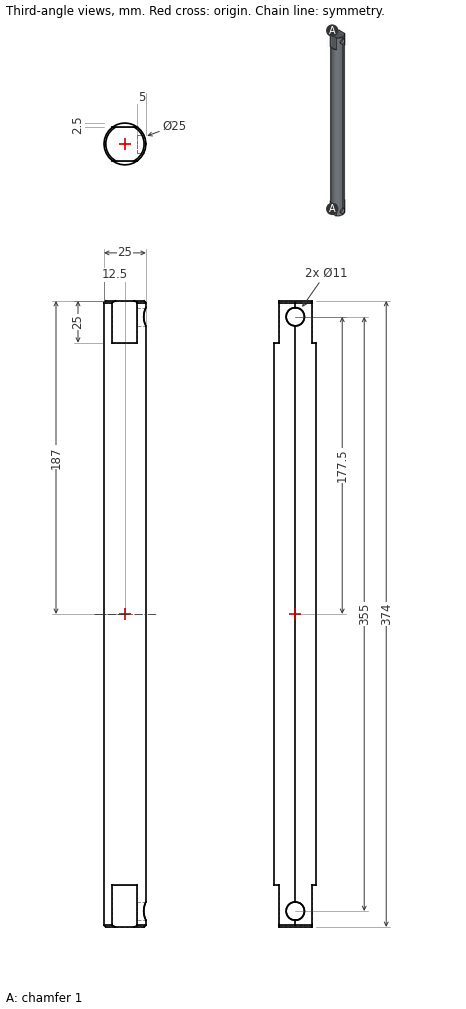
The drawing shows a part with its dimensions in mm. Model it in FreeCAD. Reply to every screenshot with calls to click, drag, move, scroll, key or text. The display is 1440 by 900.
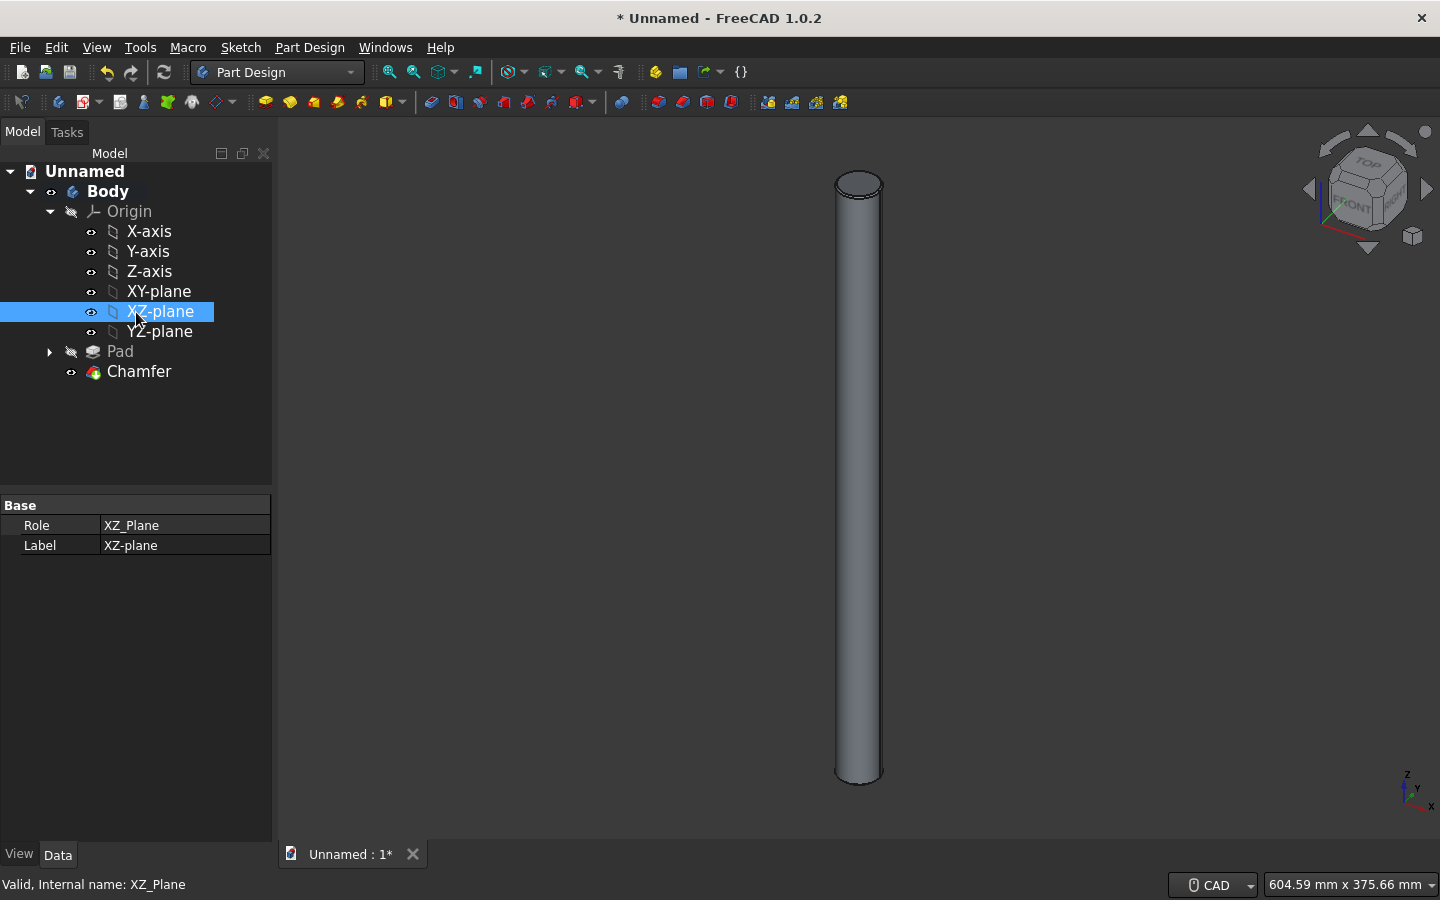
click(216, 102)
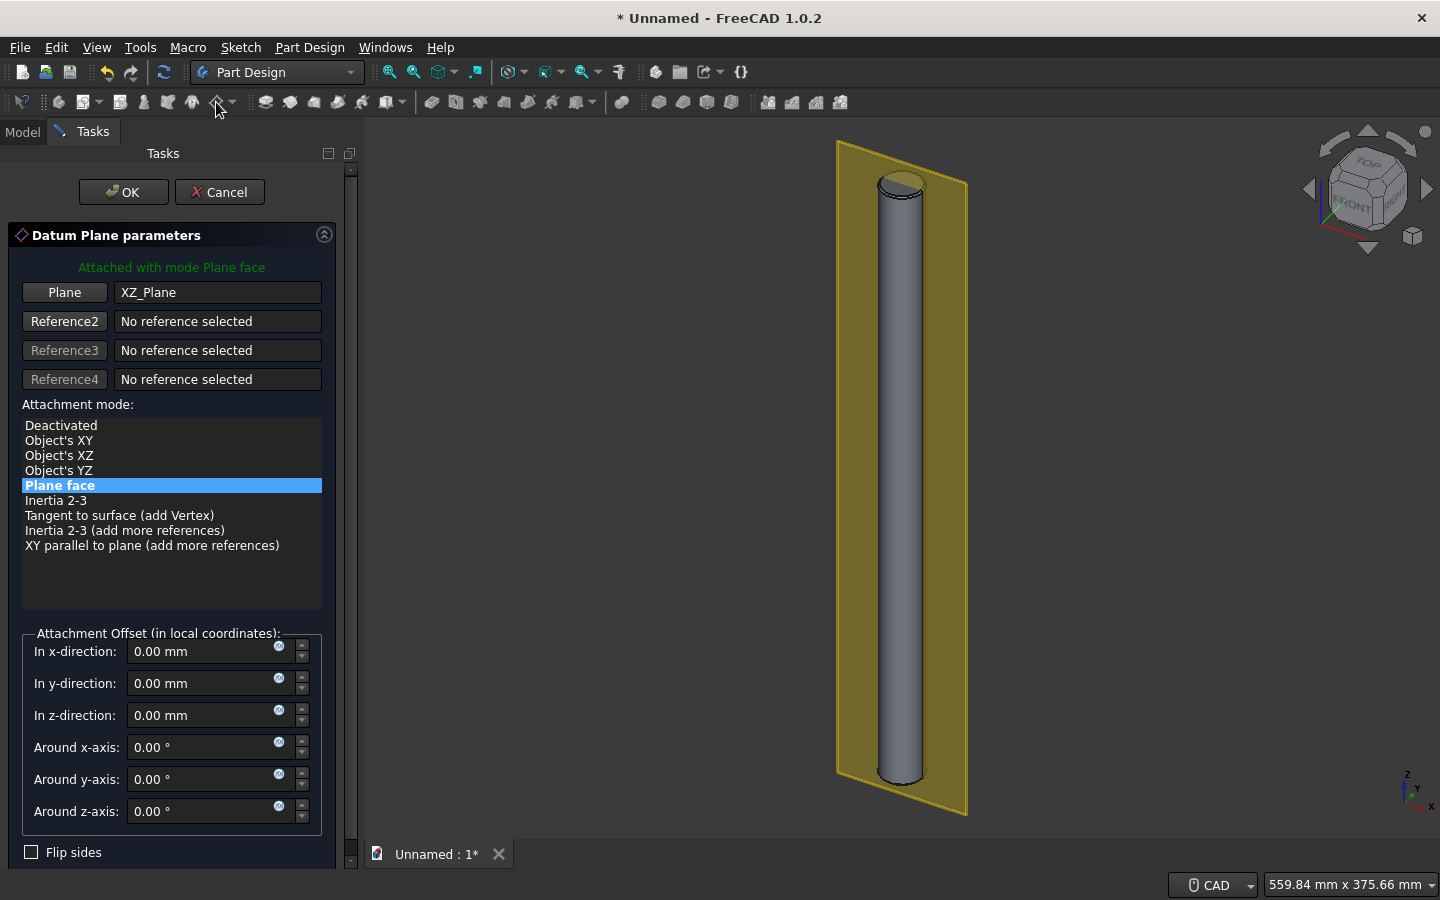
triple_click(210, 715)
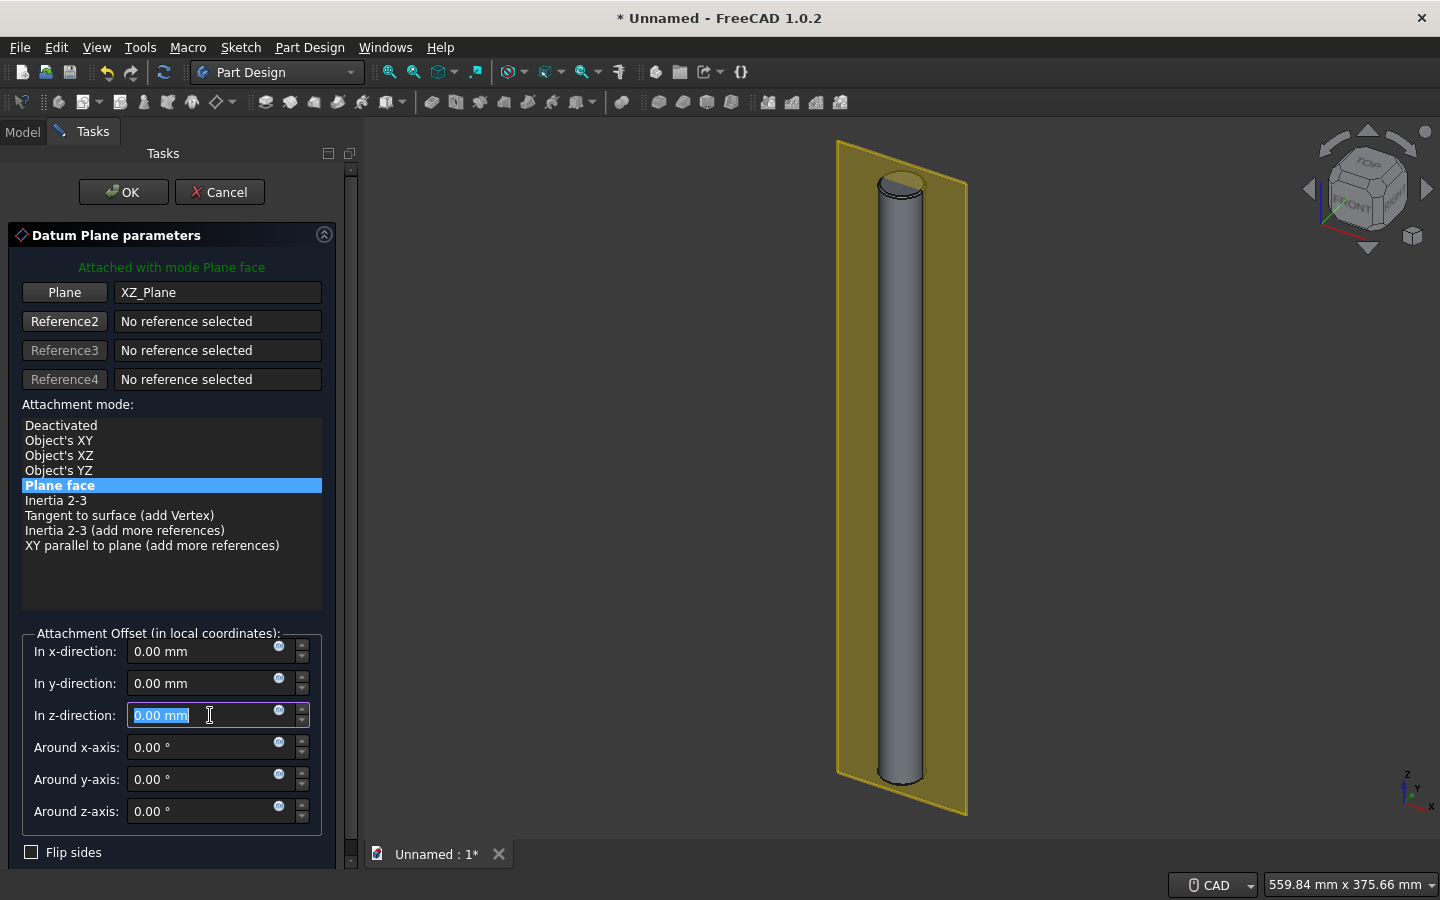
text(-12.5)
key(Tab)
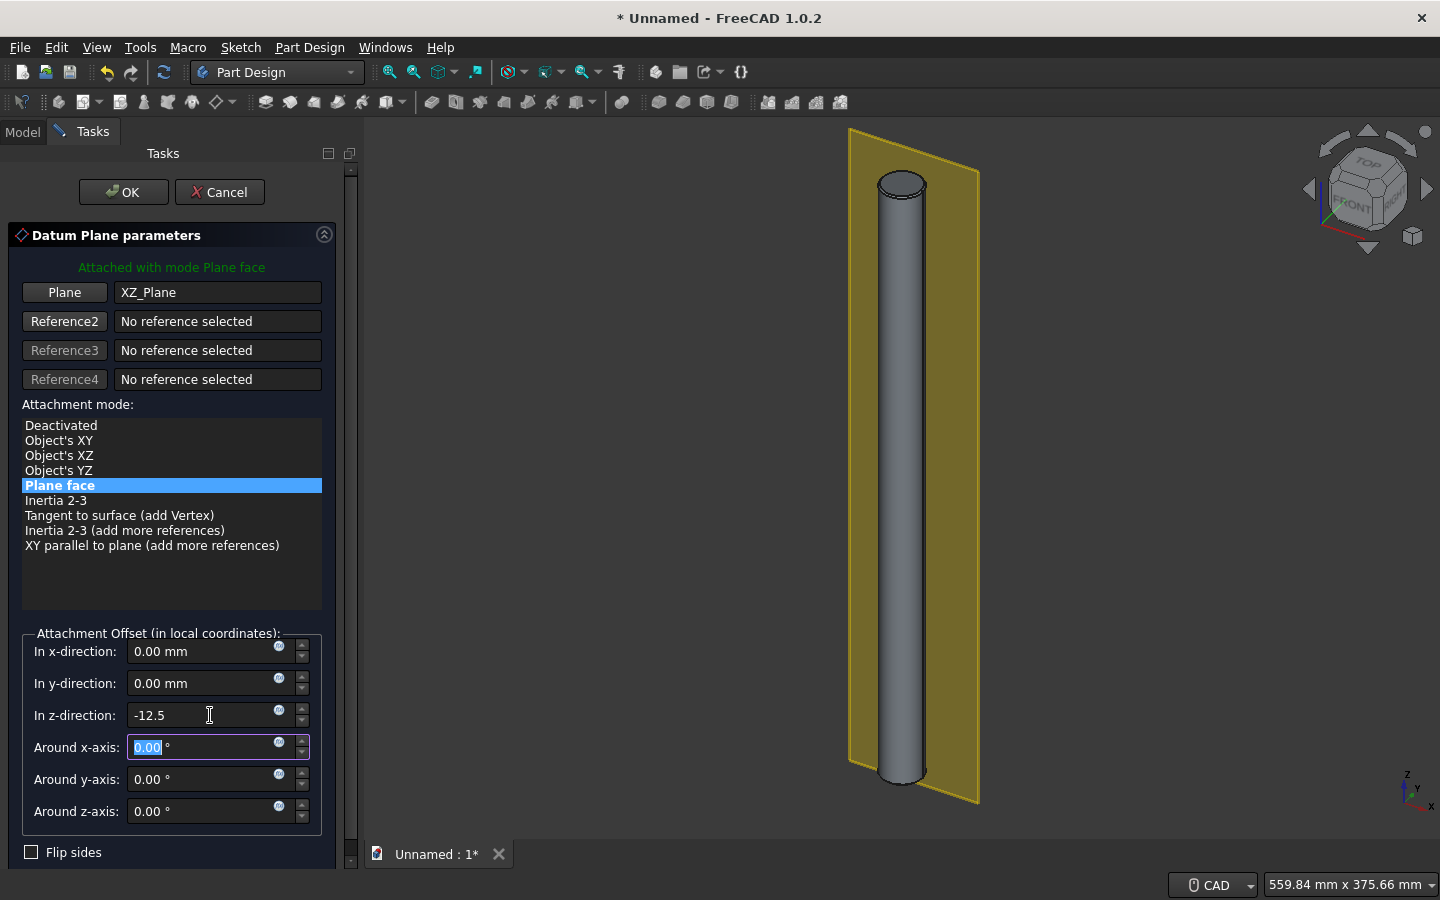
click(124, 192)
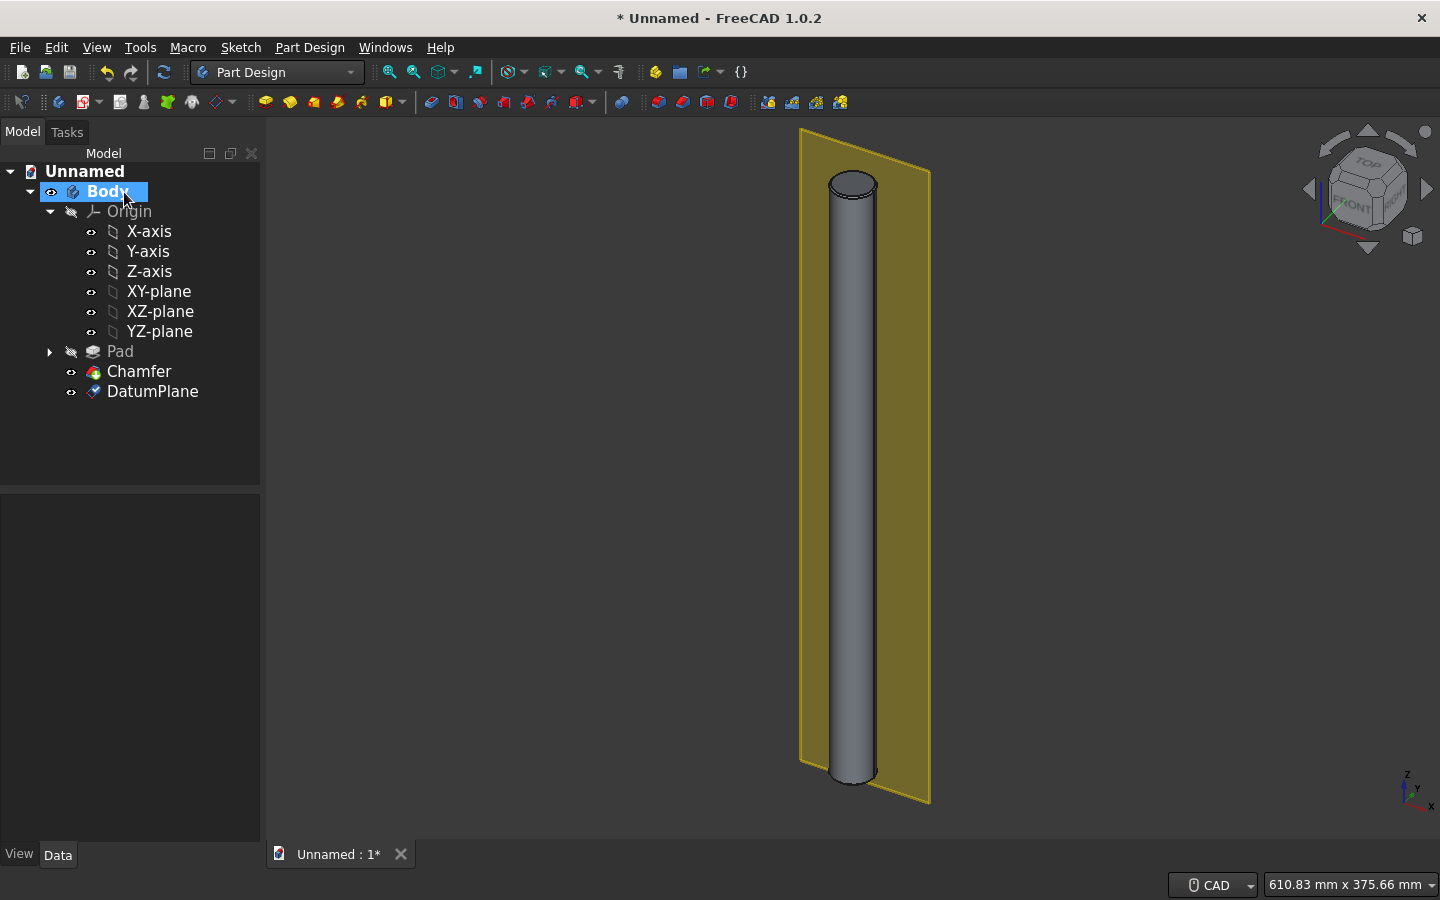
click(116, 392)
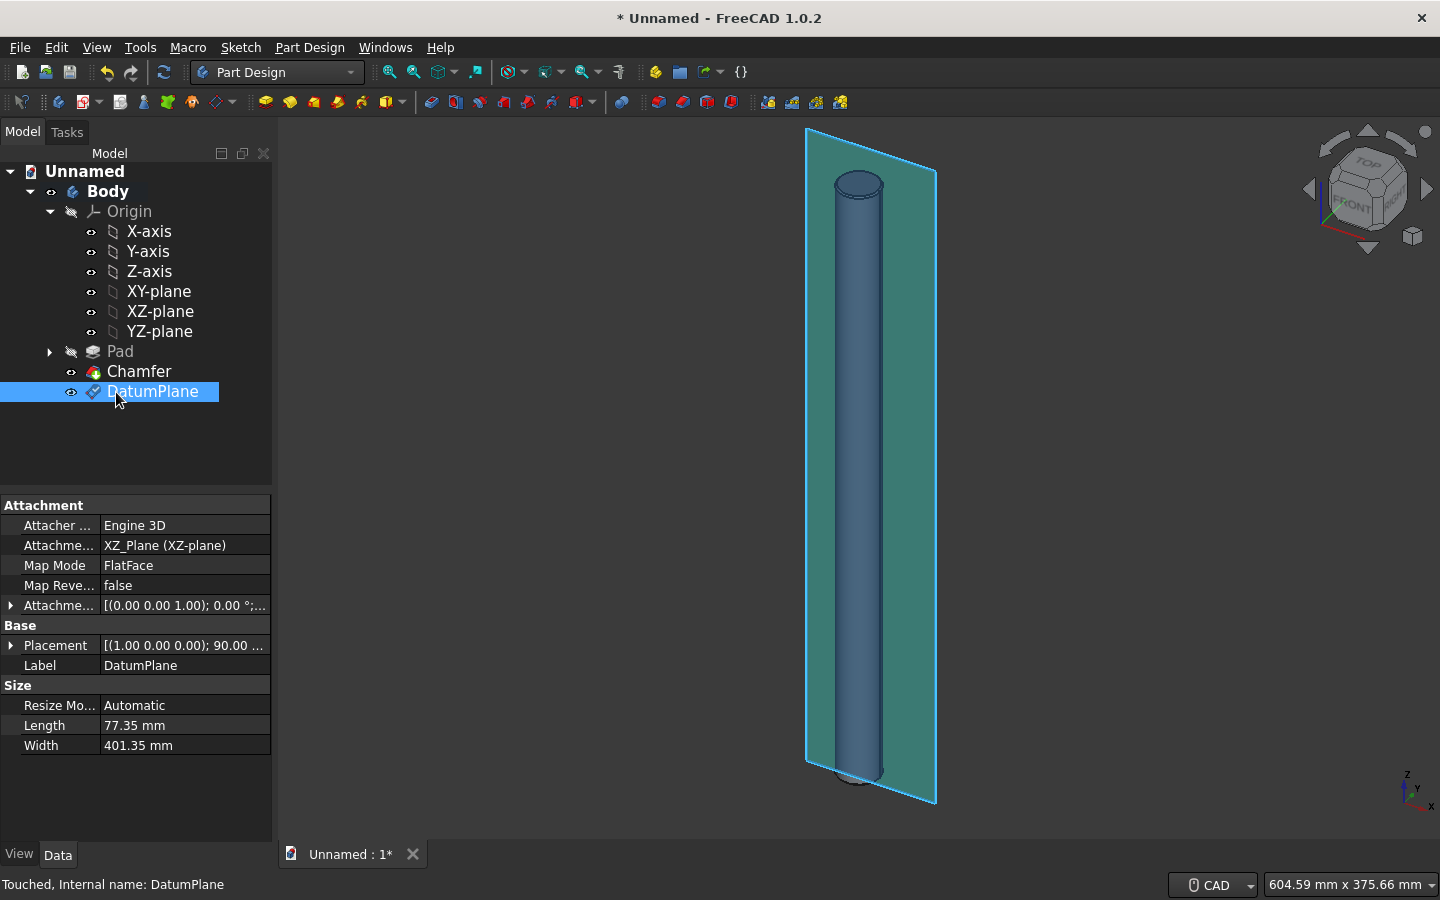
click(84, 102)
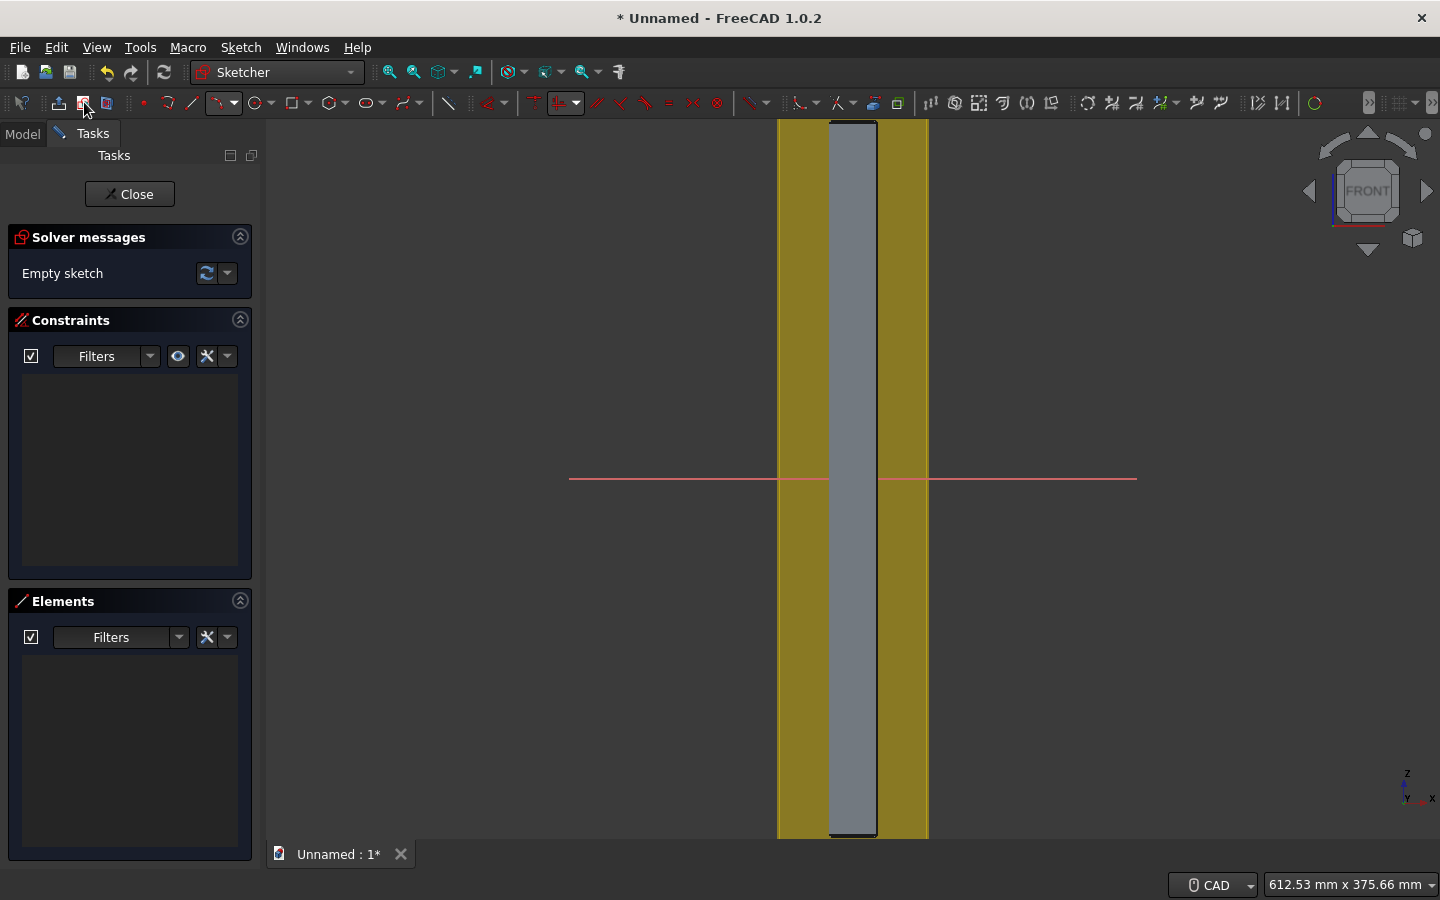
click(108, 104)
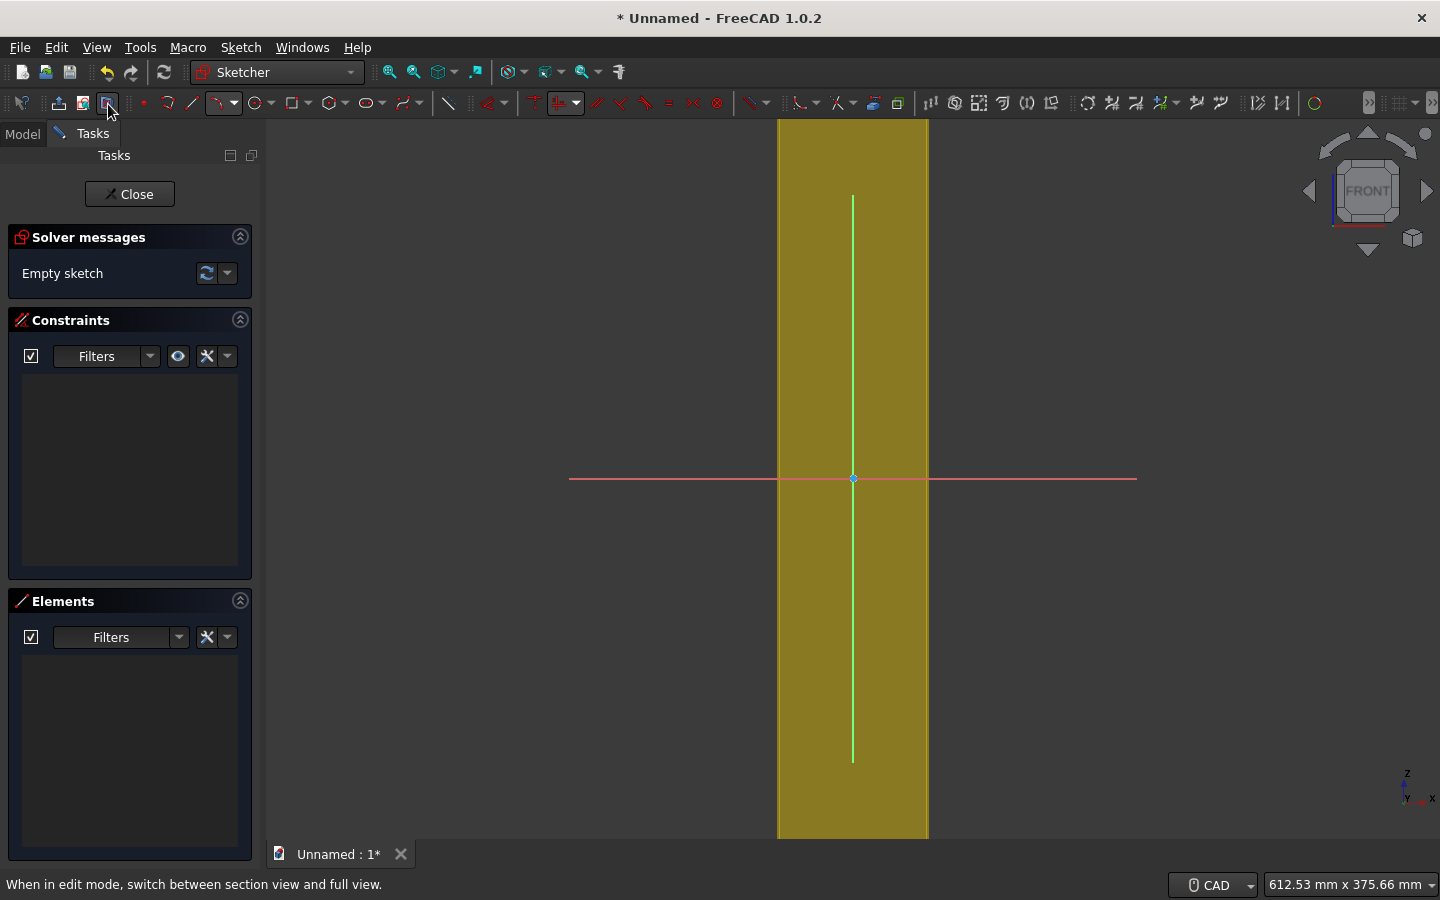
scroll(645, 479, down, 2)